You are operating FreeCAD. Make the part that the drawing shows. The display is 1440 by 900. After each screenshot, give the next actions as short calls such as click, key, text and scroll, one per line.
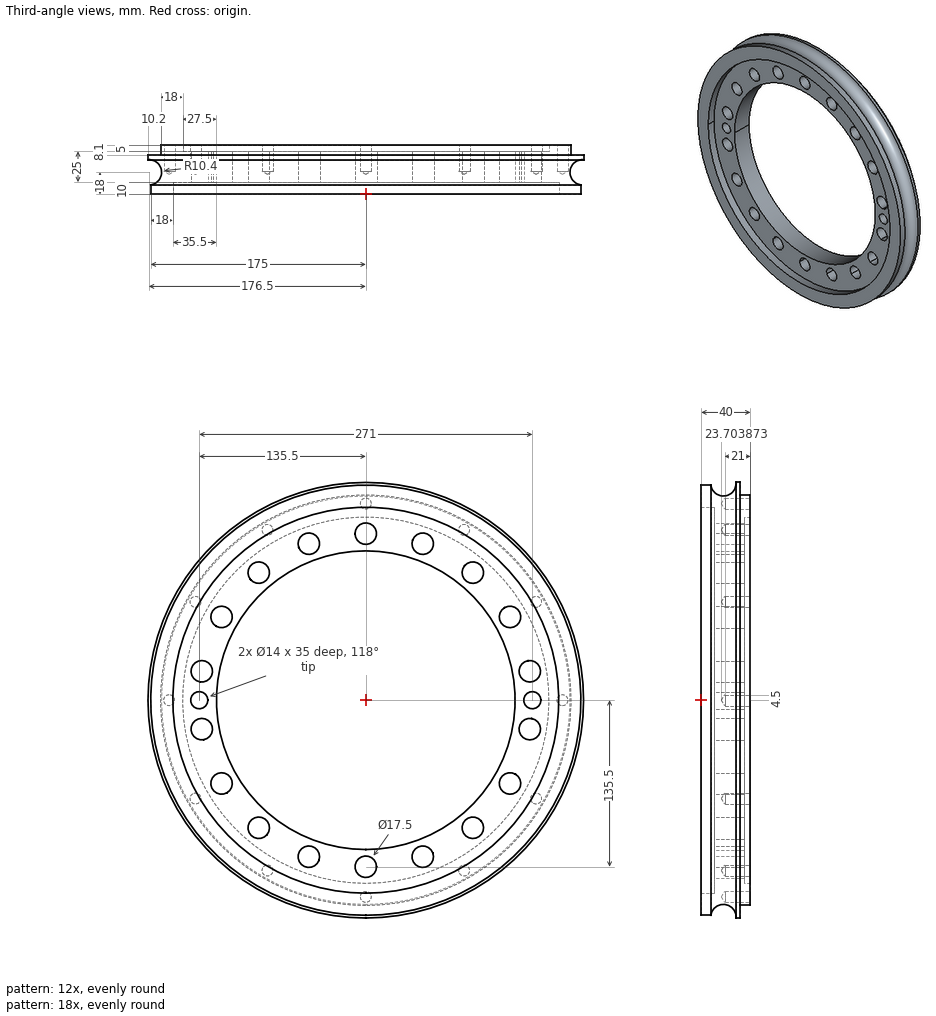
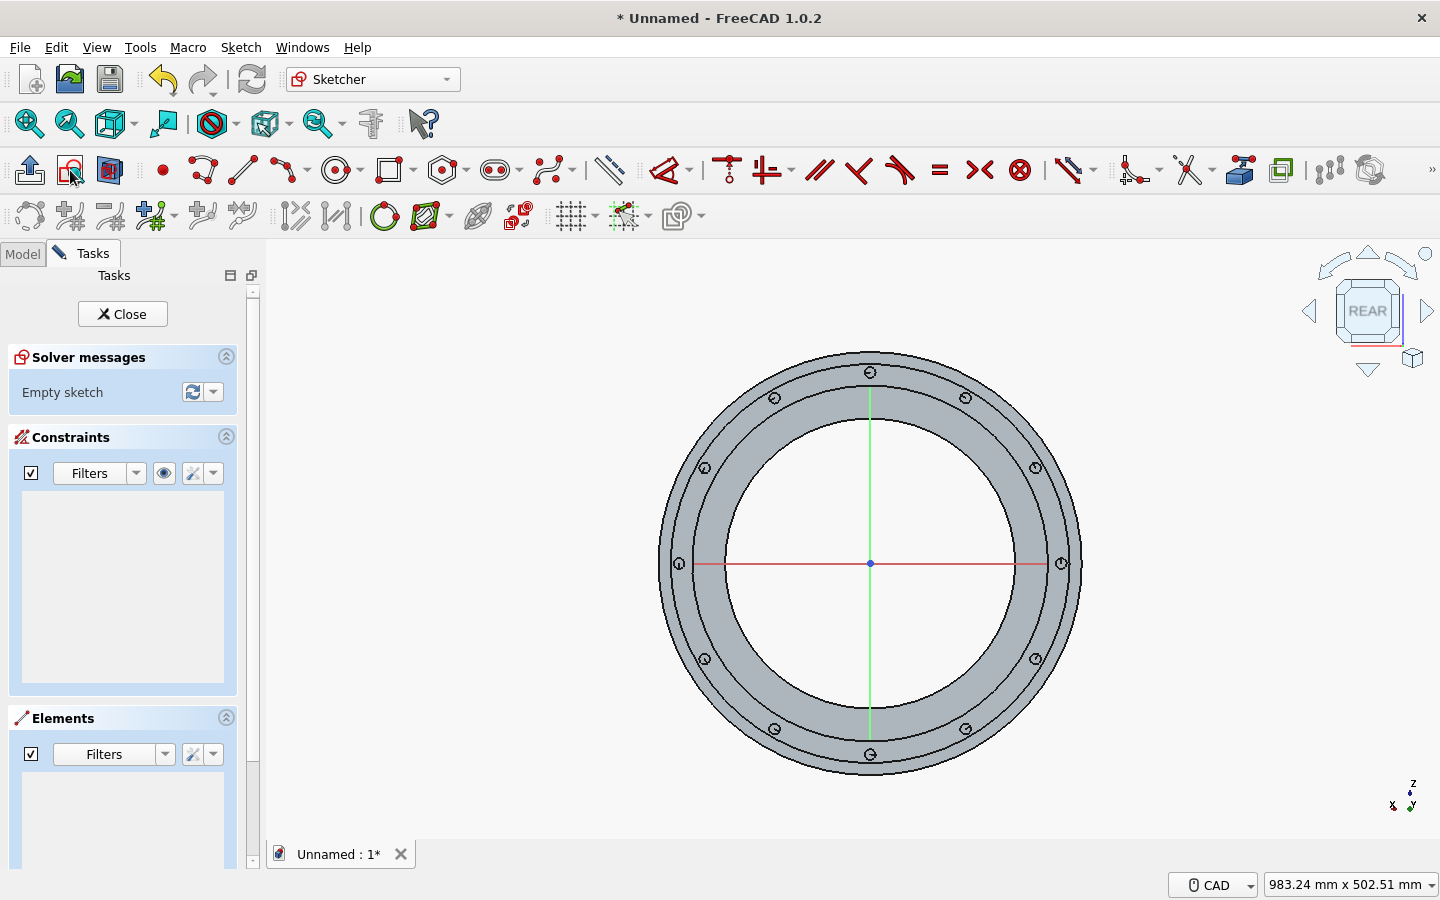
scroll(875, 735, up, 15)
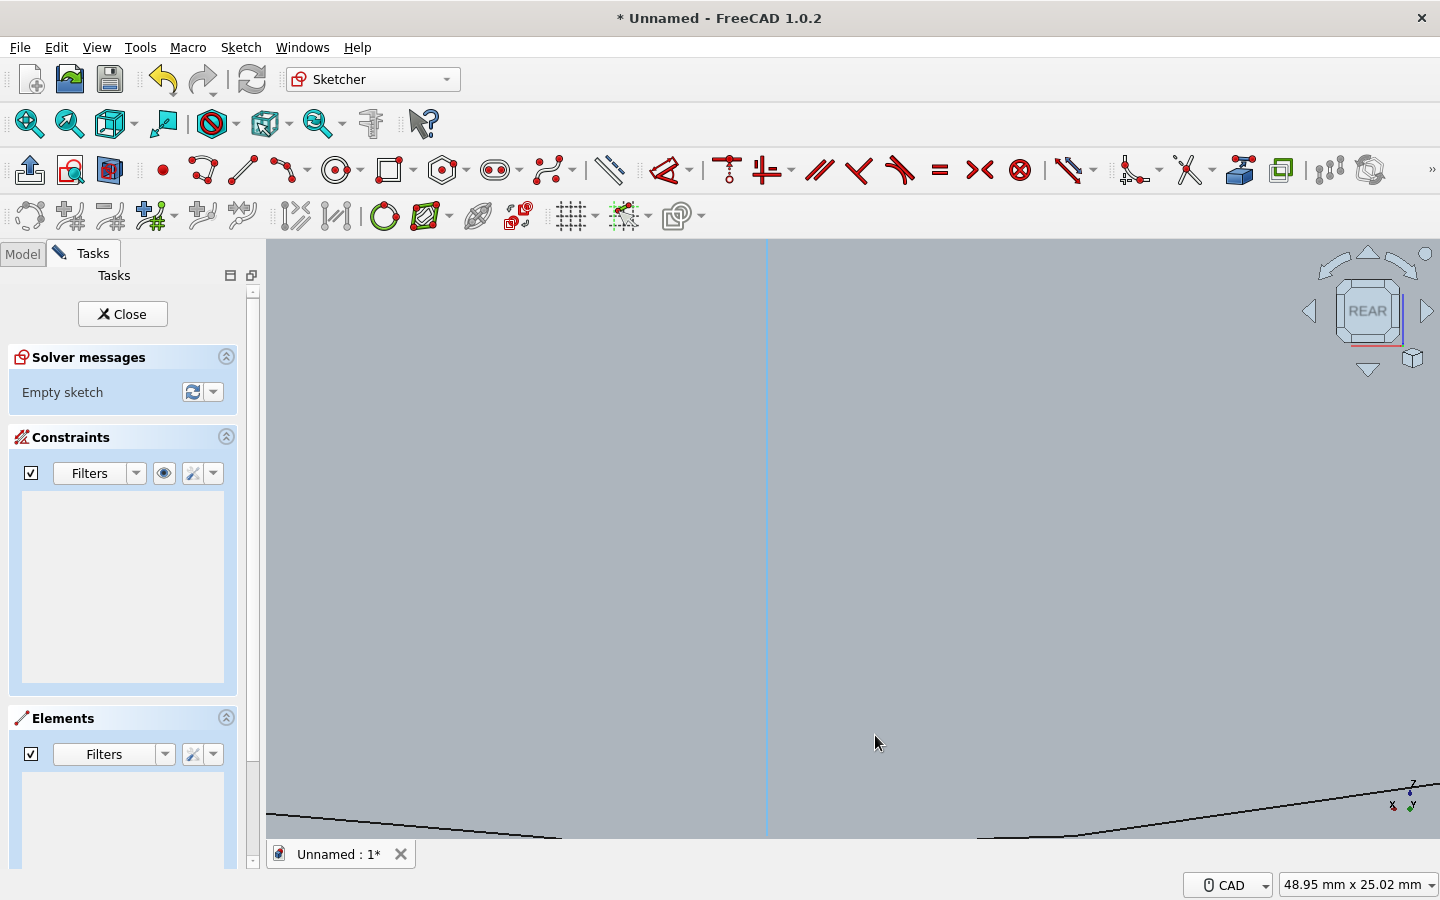
click(336, 170)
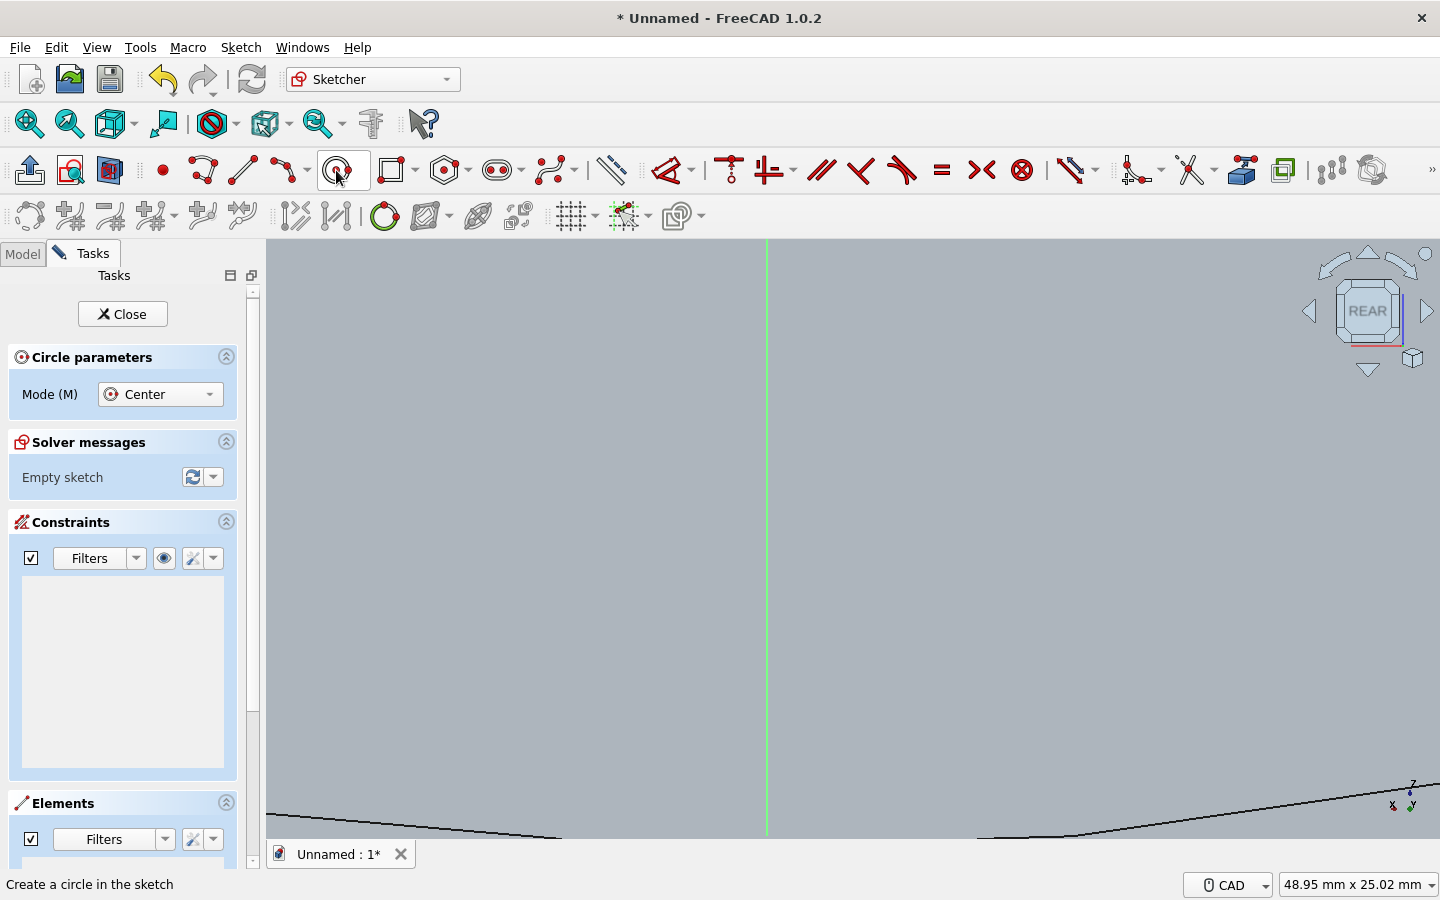
click(767, 526)
move(916, 377)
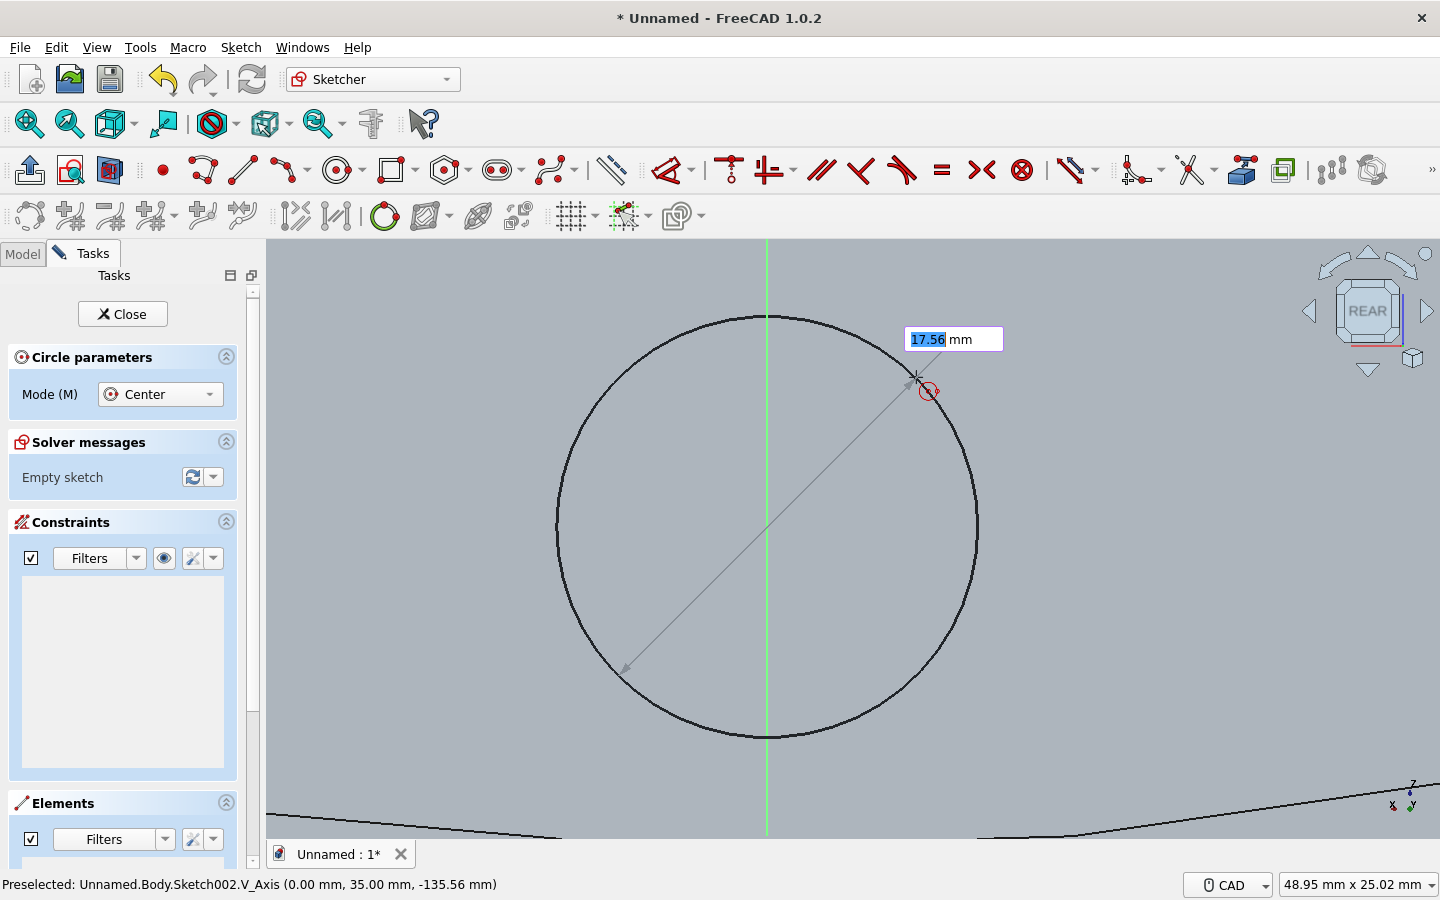
text(17.5)
key(Return)
key(Escape)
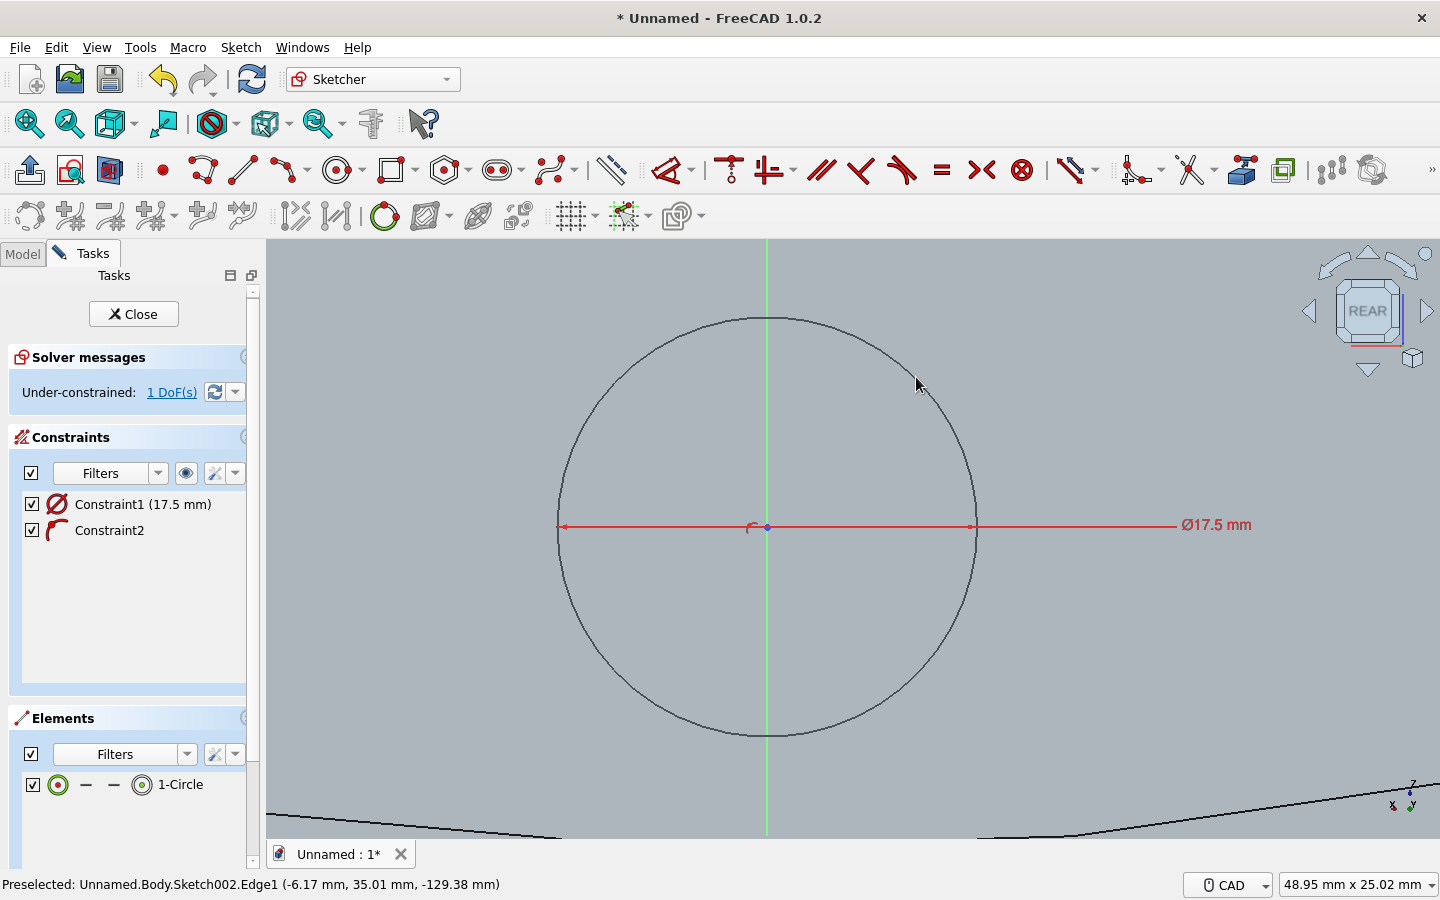
click(666, 170)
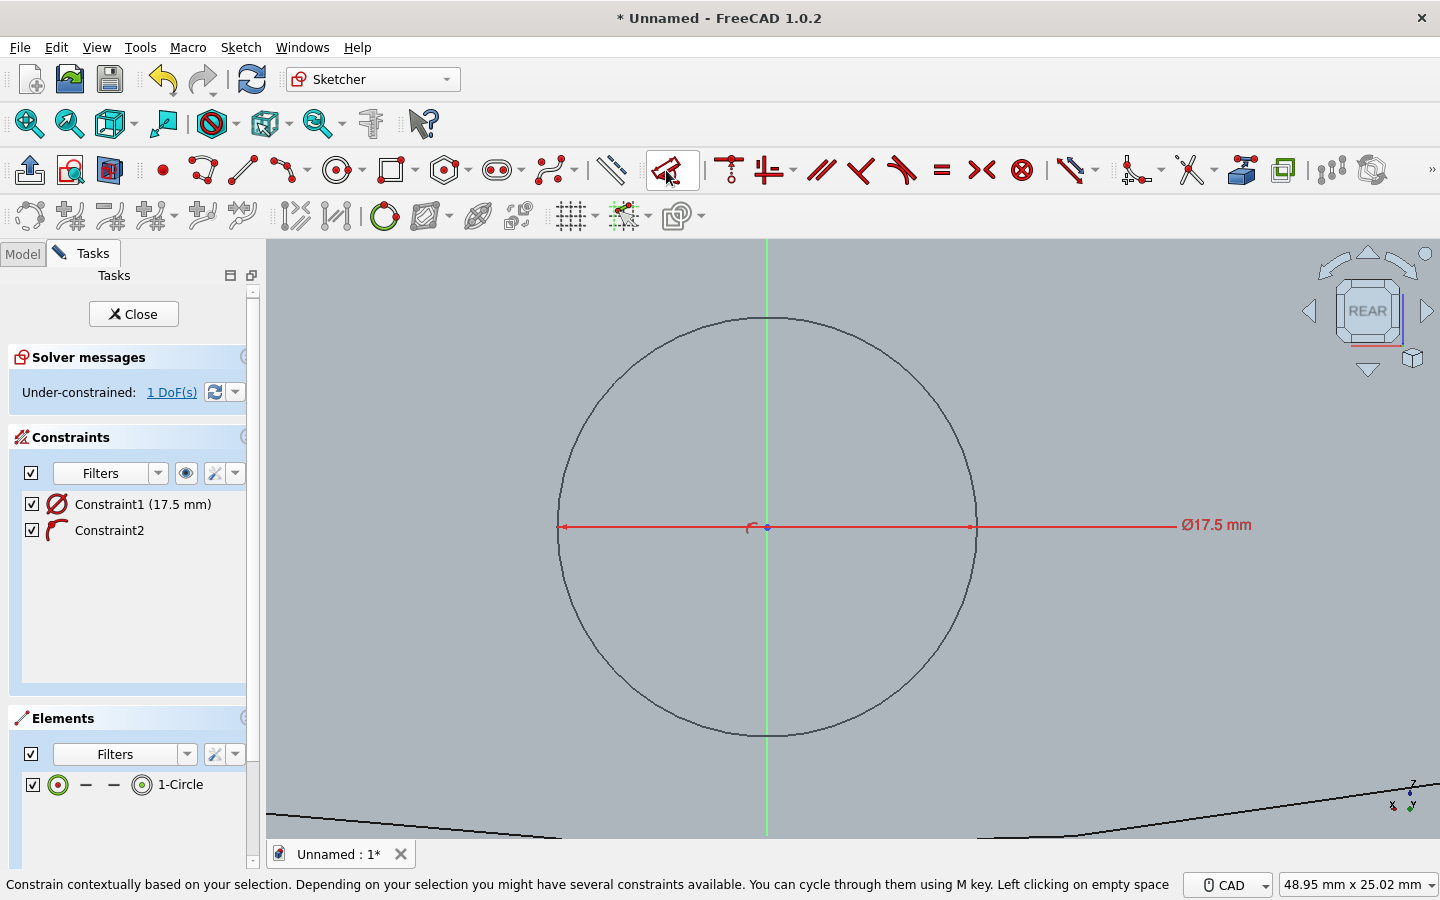
click(767, 527)
click(801, 397)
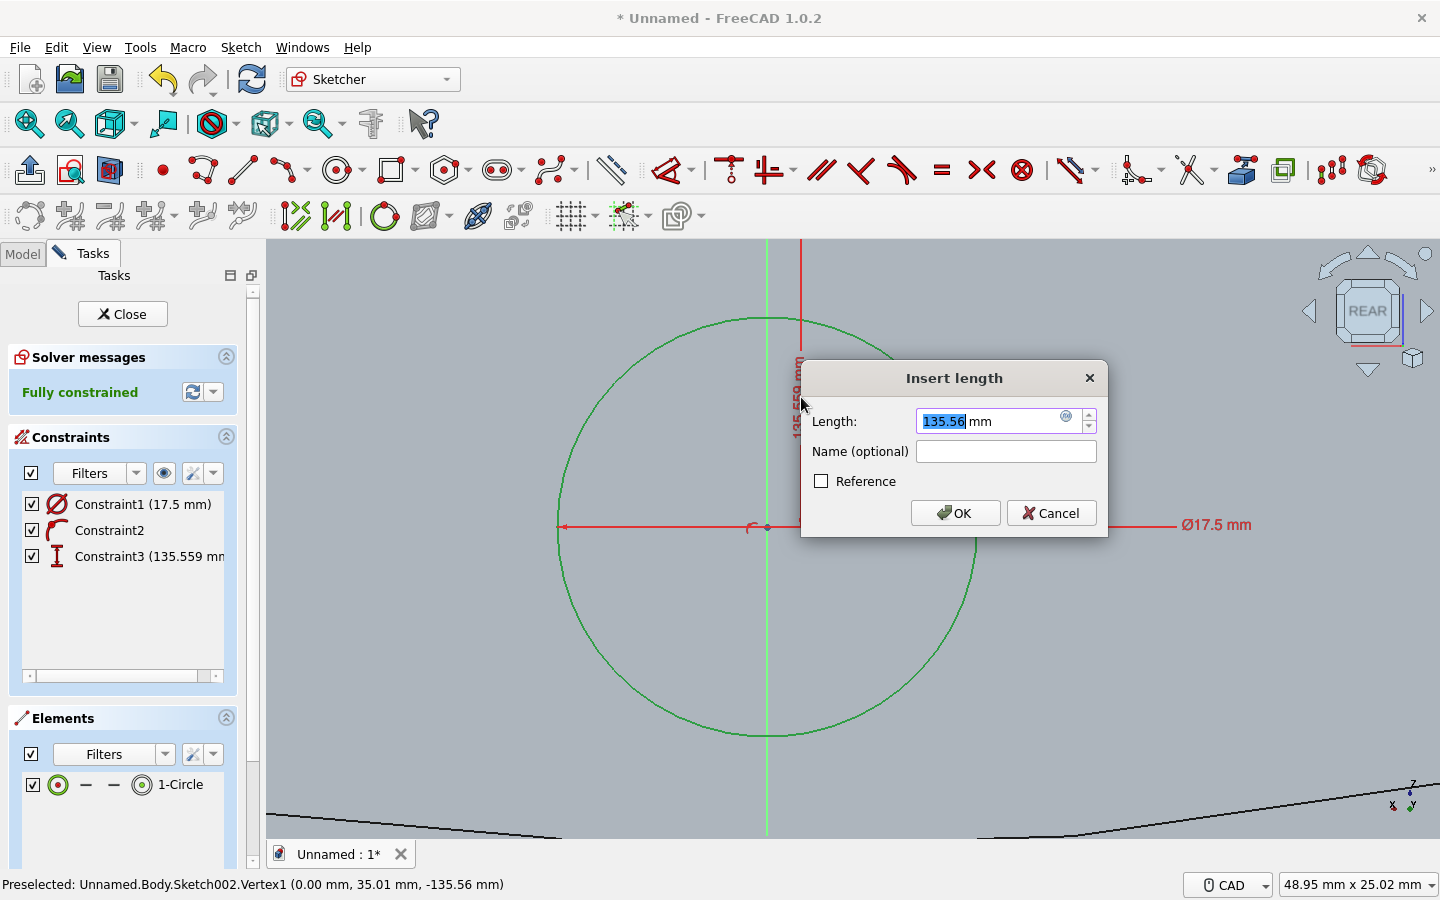
text(135.5)
key(Return)
key(Escape)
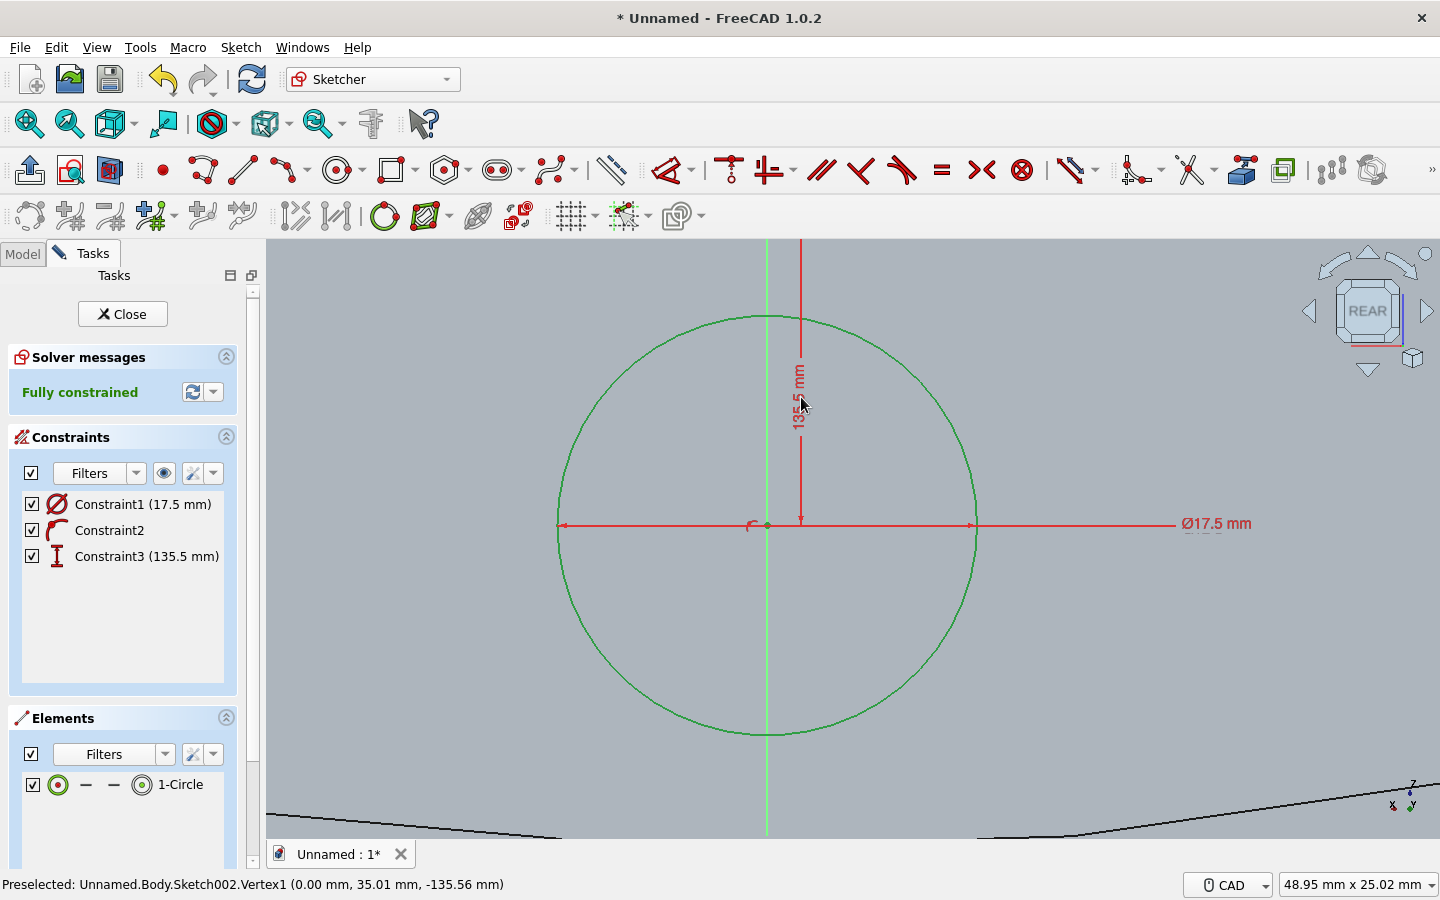
click(123, 314)